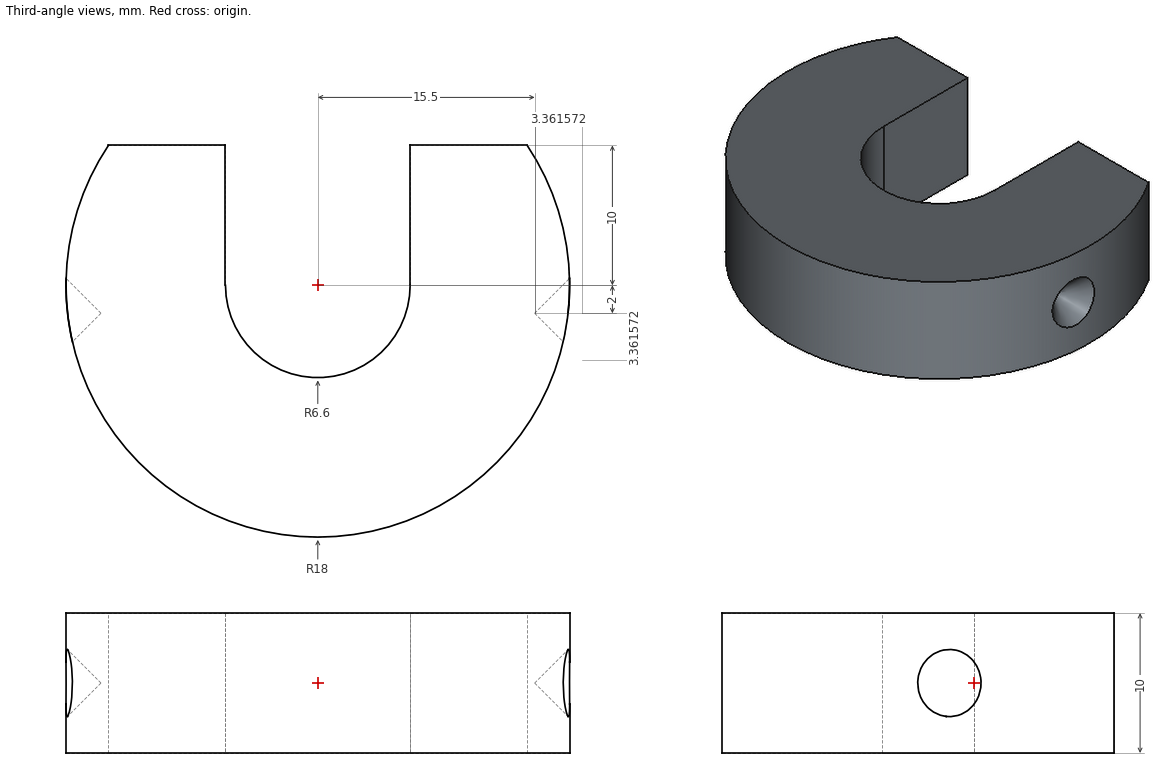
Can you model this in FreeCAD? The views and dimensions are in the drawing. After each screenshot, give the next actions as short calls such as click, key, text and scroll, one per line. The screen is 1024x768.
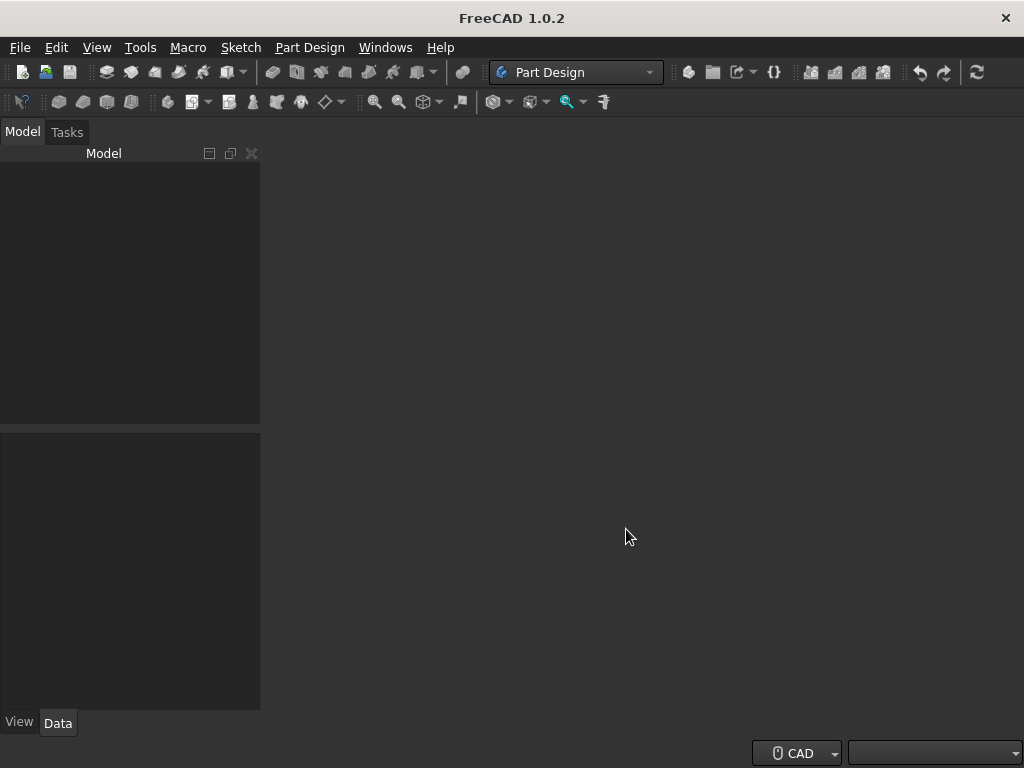
key(ctrl+n)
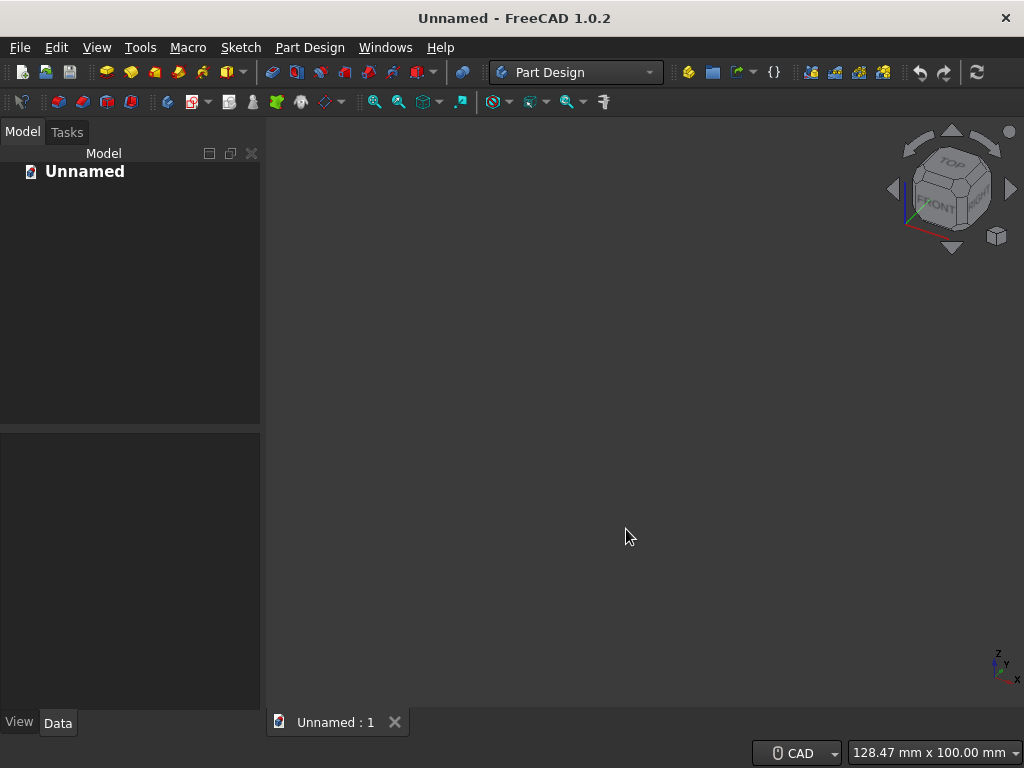
click(192, 102)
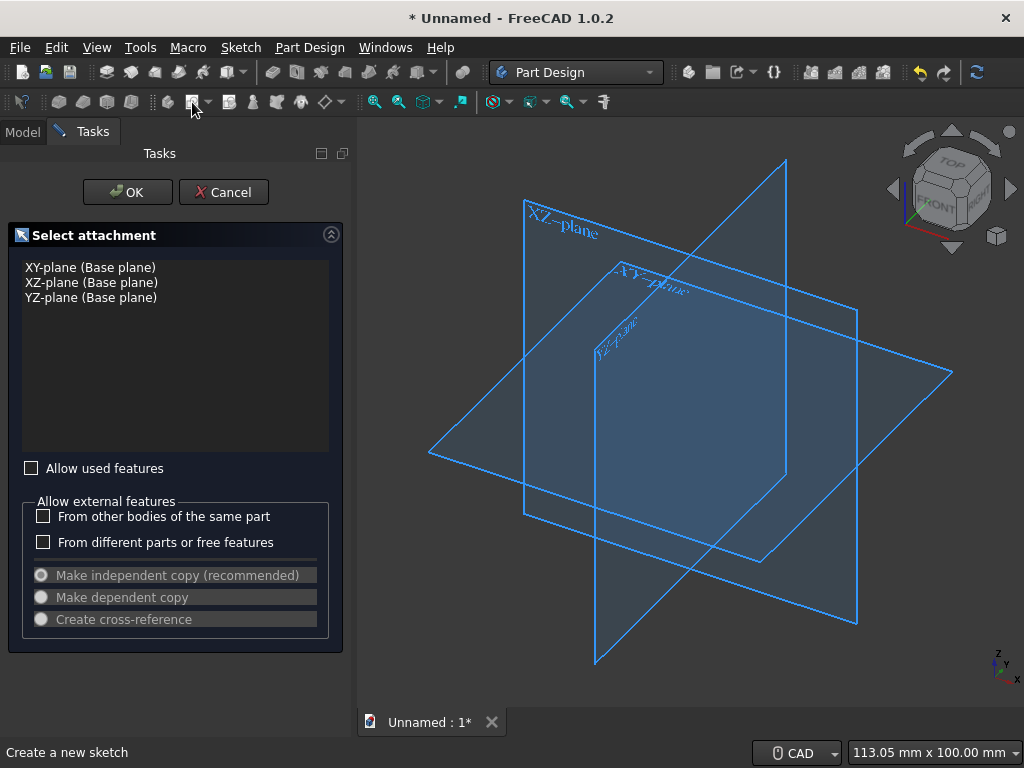
click(82, 268)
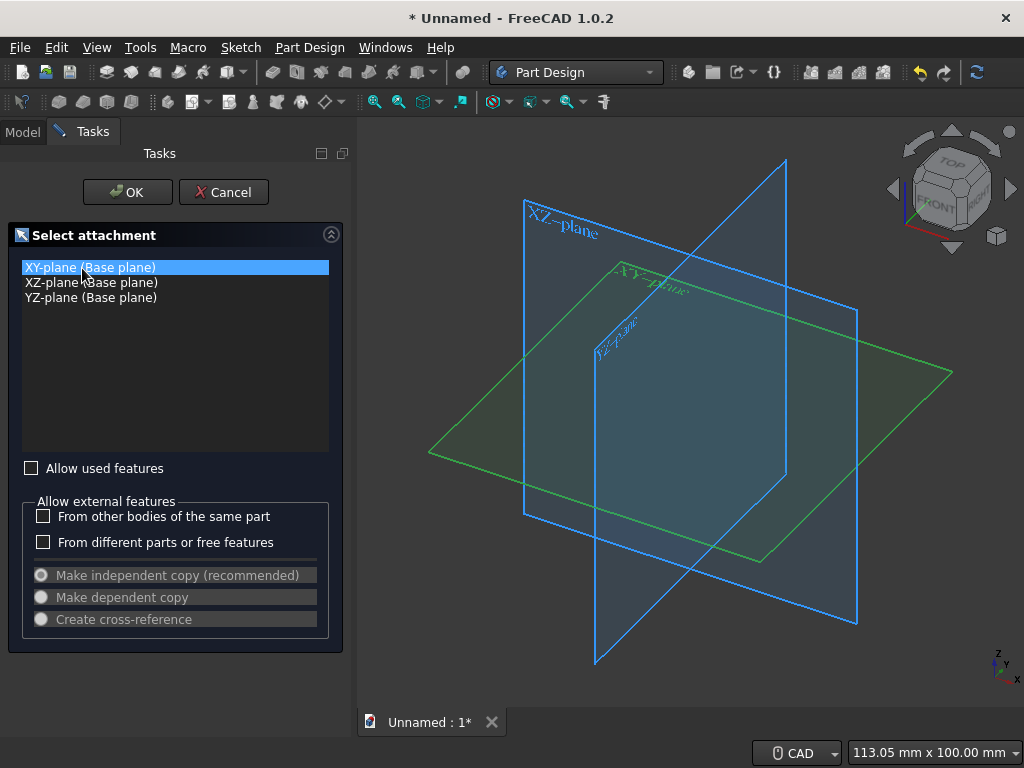
click(128, 192)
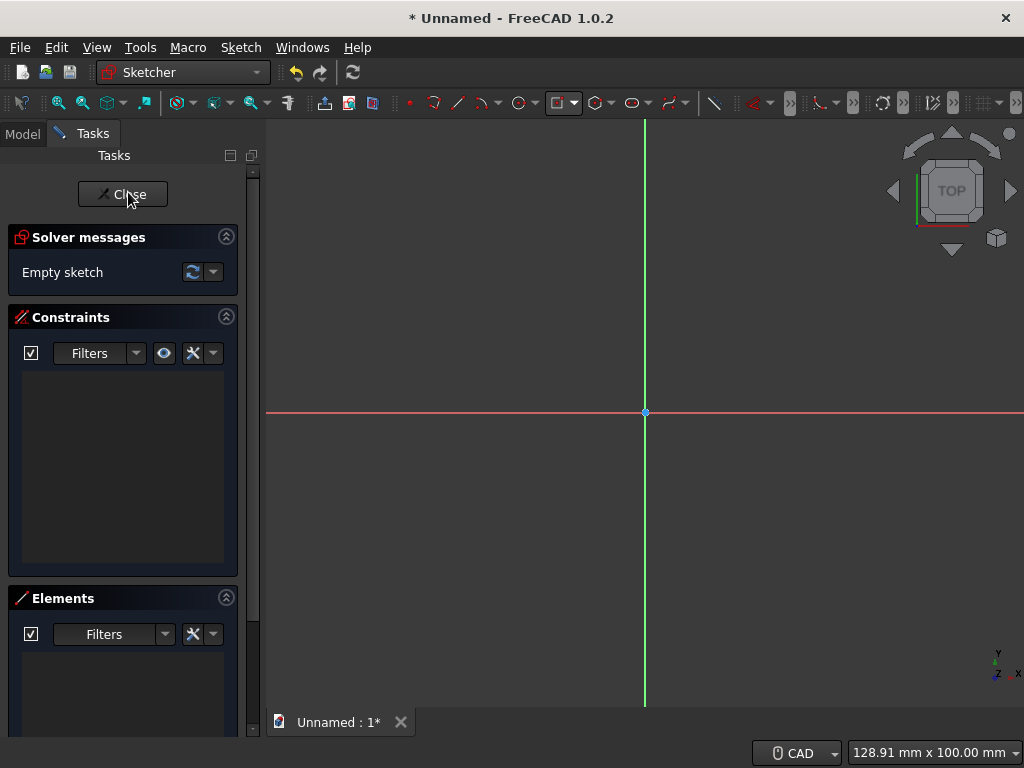
scroll(701, 456, up, 4)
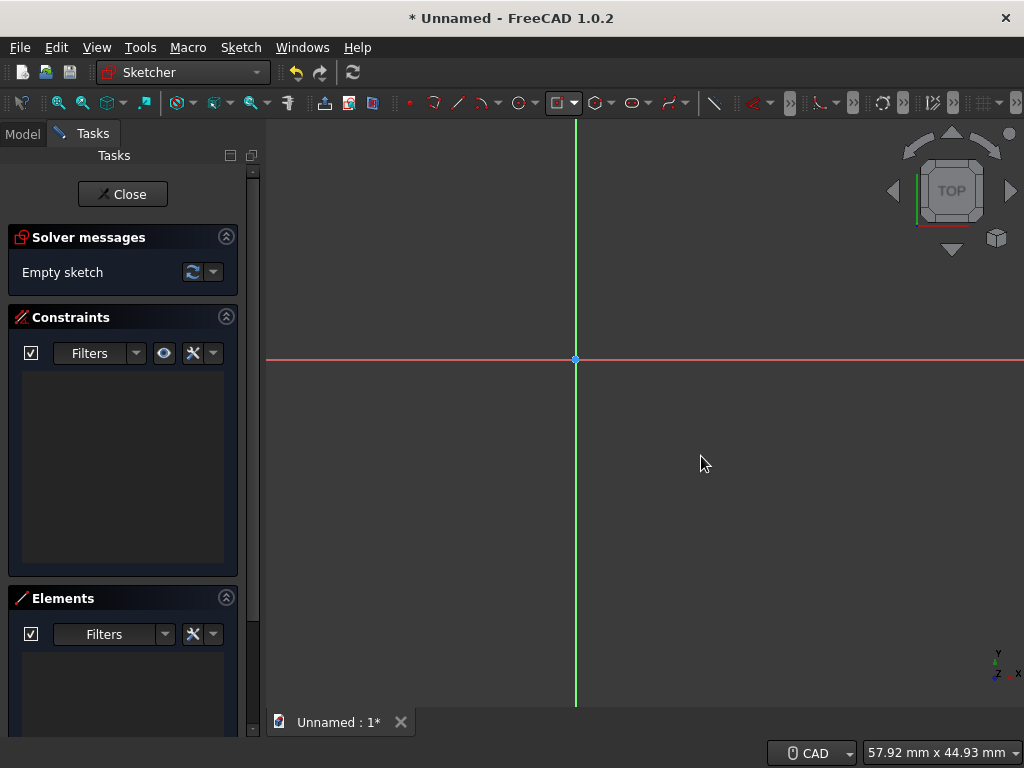
key(g)
key(m)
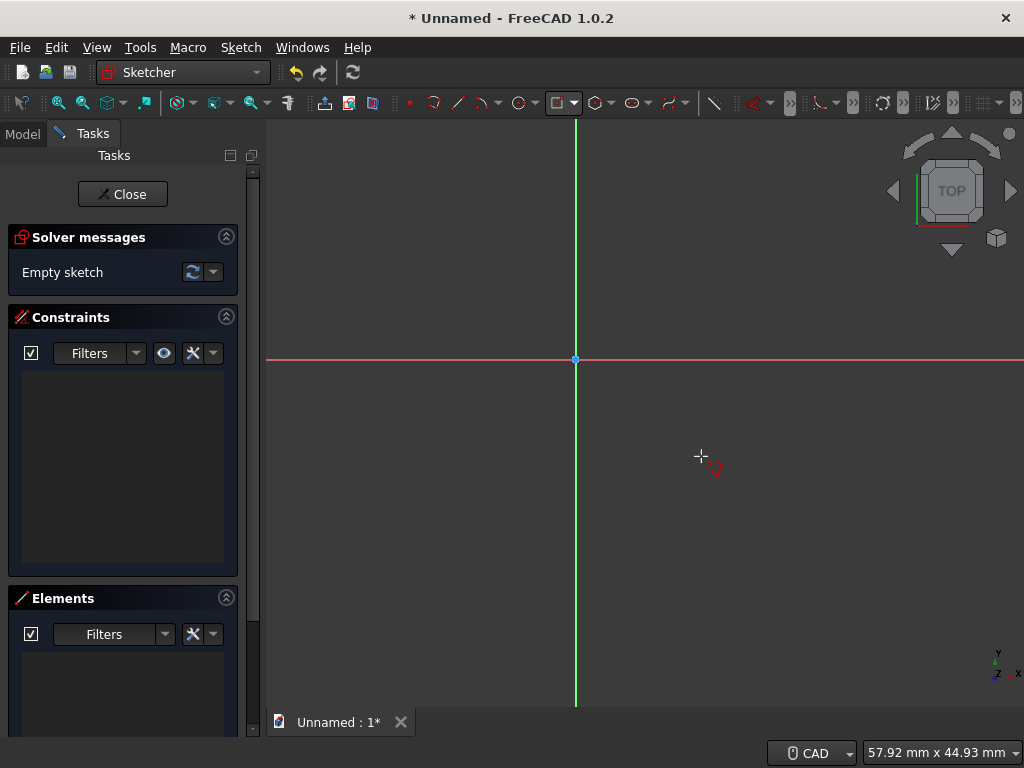
click(772, 229)
click(662, 229)
click(662, 360)
right_click(662, 360)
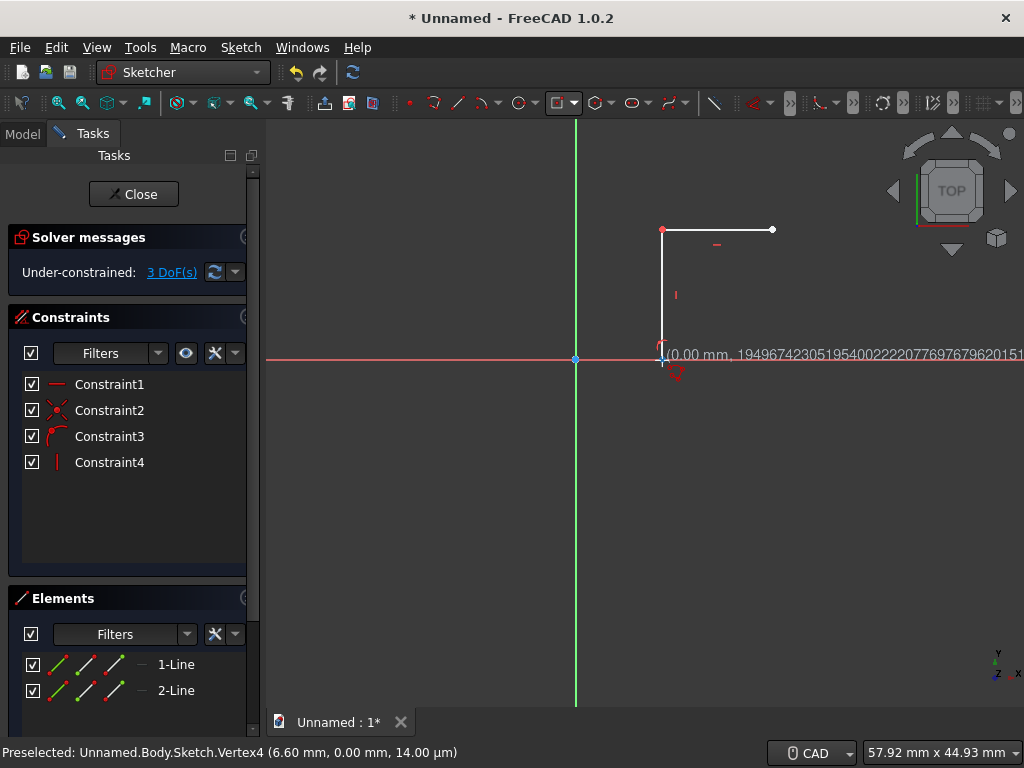
click(489, 360)
click(489, 229)
click(380, 229)
right_click(380, 229)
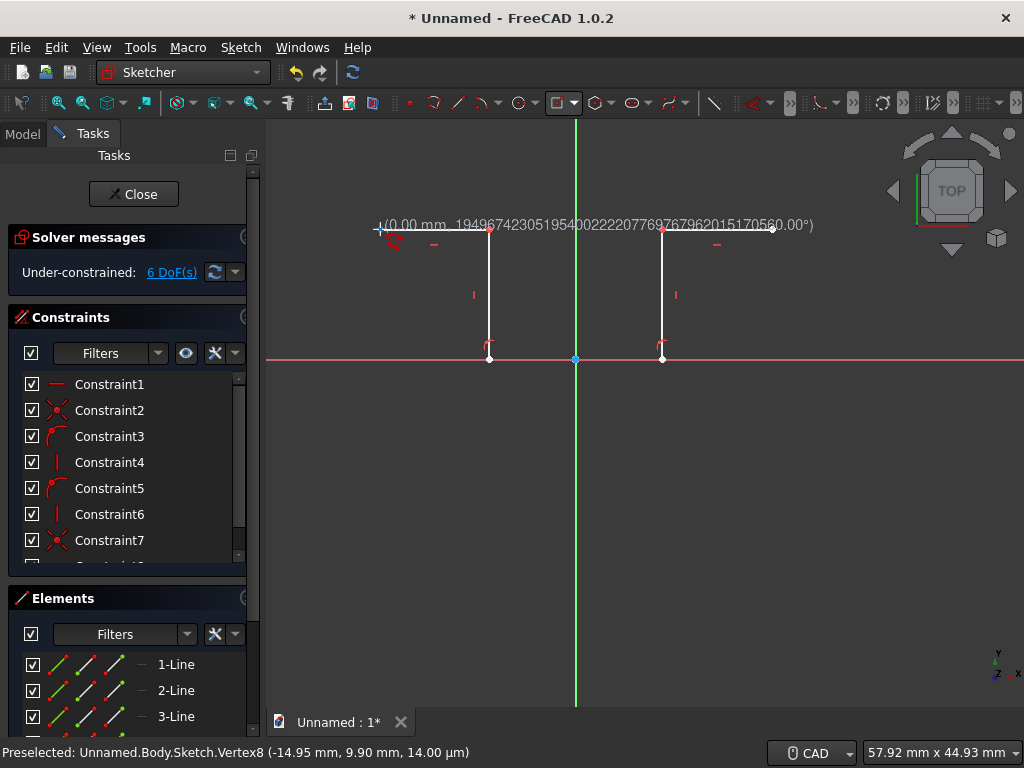
key(g)
key(3)
key(a)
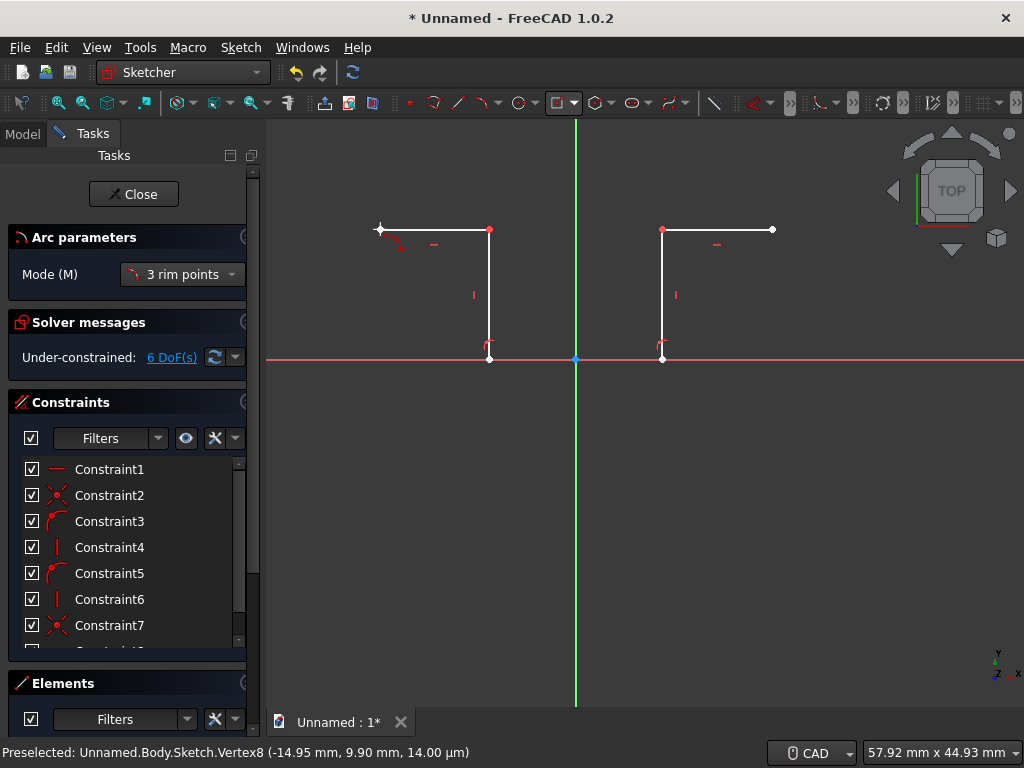
click(662, 360)
click(489, 360)
click(549, 442)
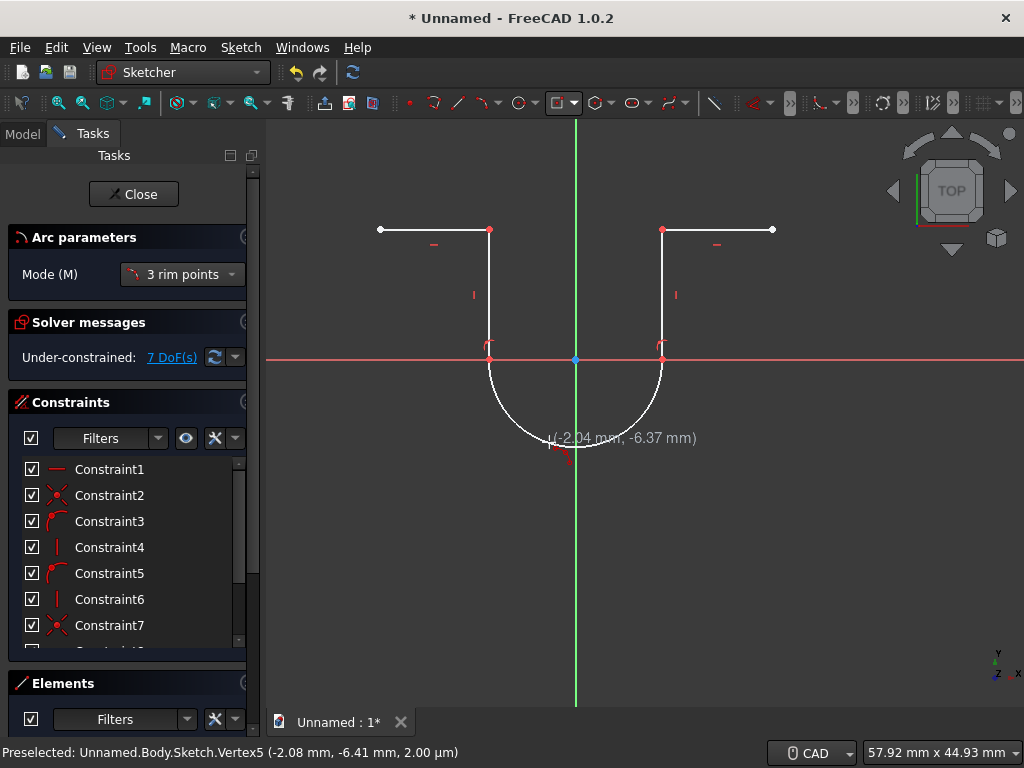
click(380, 230)
click(772, 230)
click(477, 574)
key(Escape)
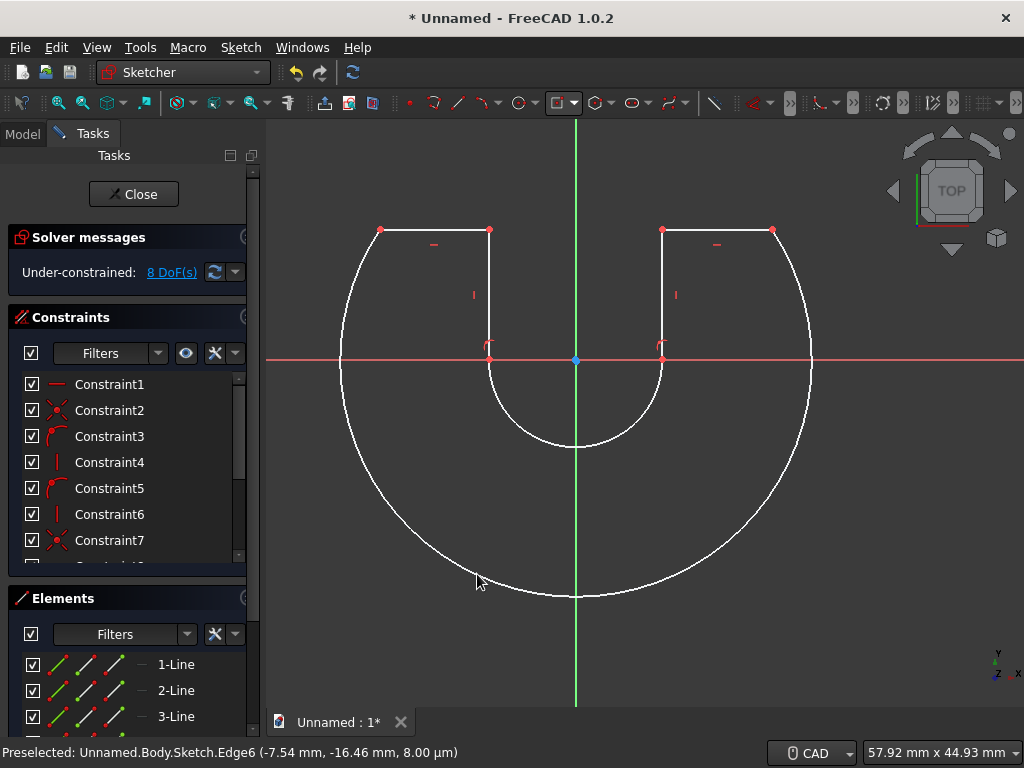
click(662, 269)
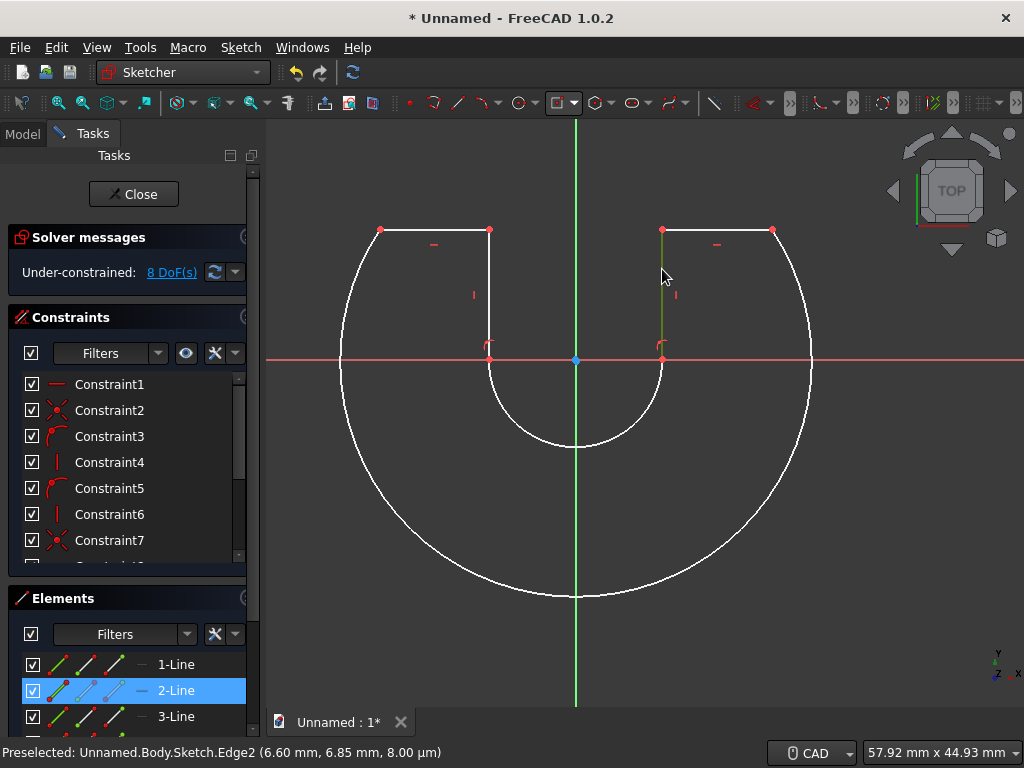
click(524, 430)